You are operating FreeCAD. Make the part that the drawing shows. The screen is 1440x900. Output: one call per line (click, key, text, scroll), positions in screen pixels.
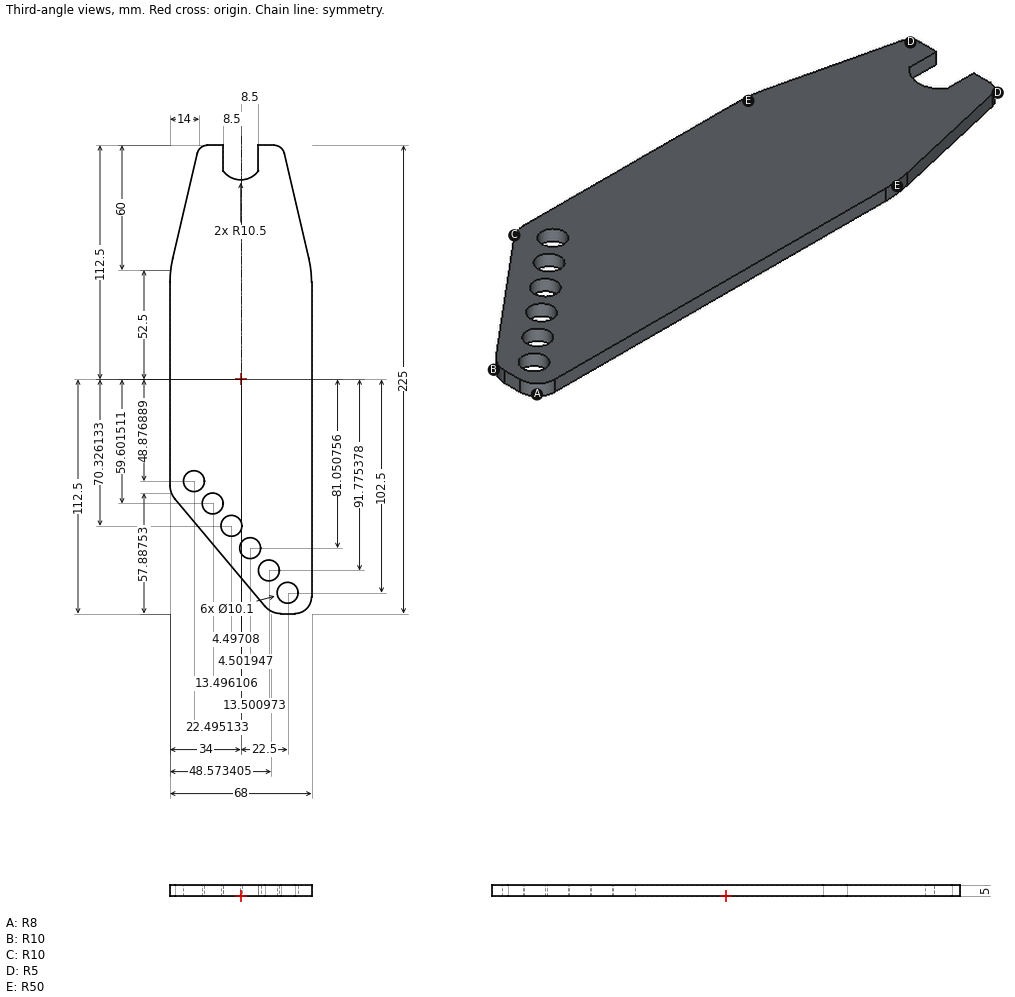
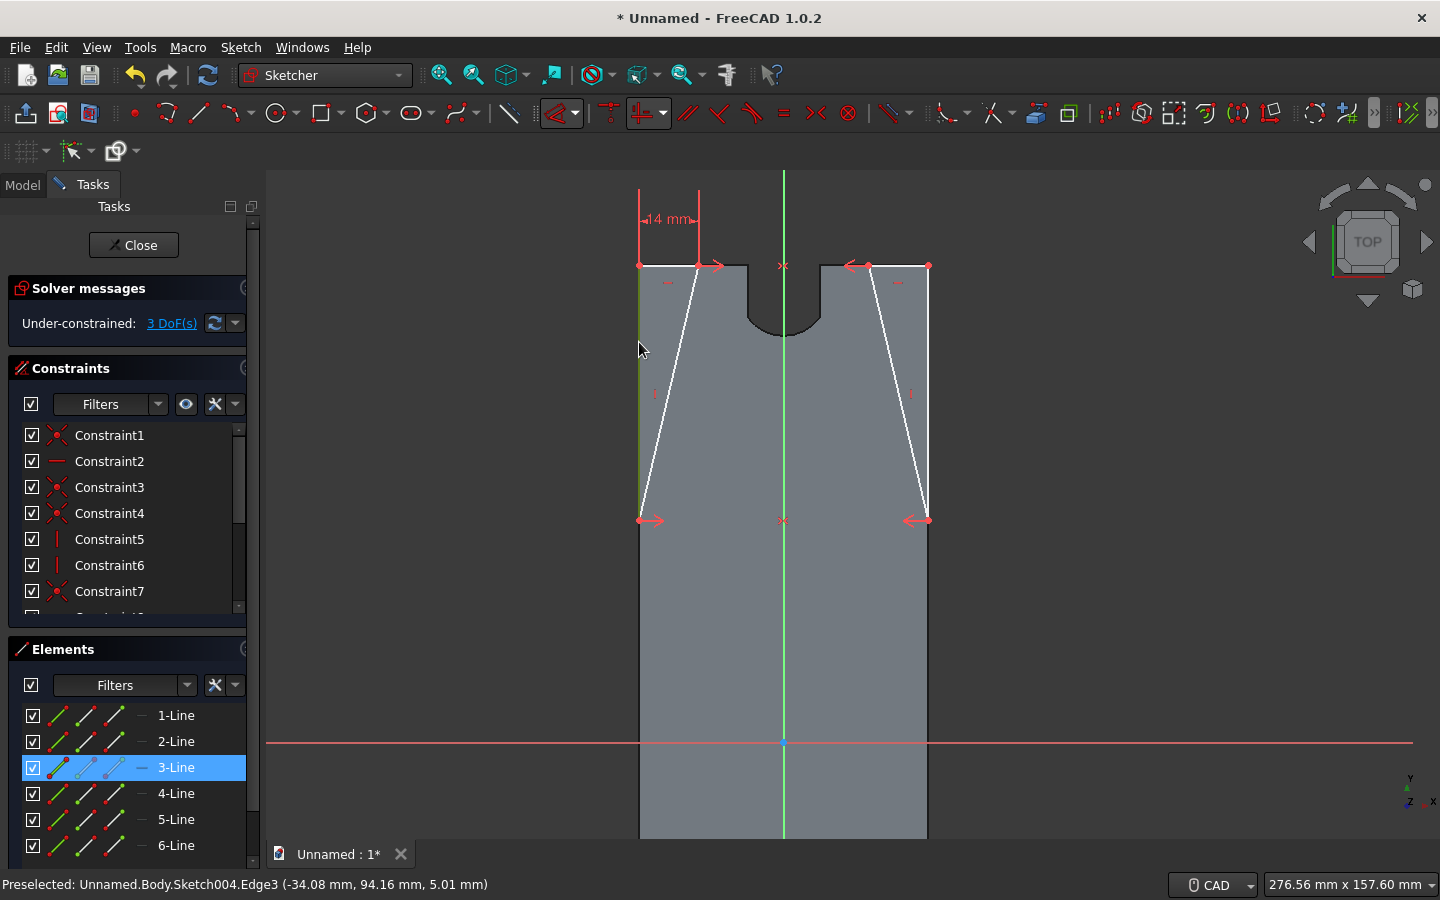
key(i)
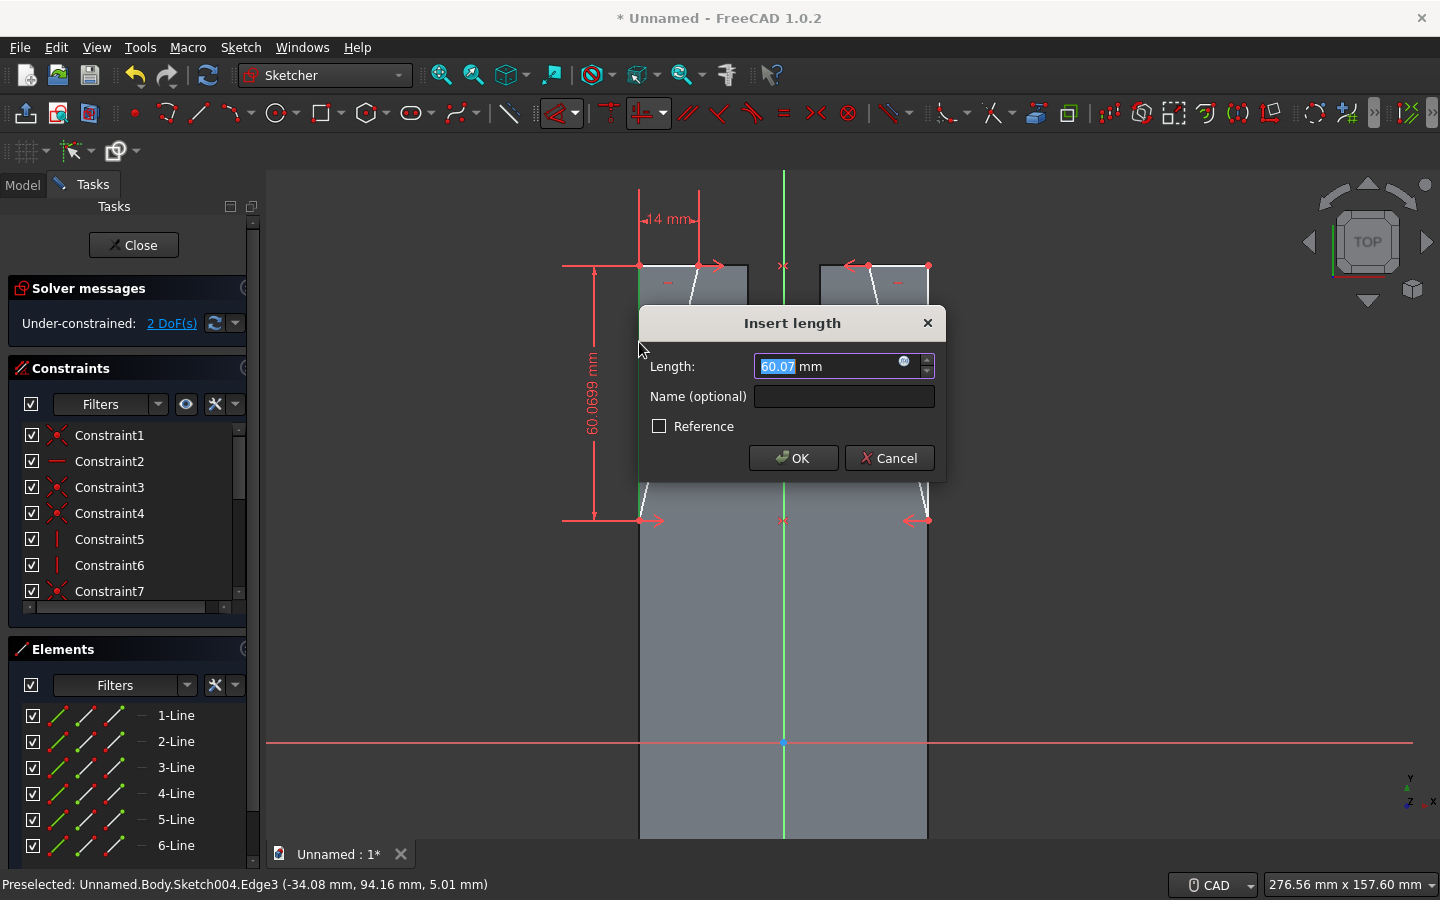
text(60)
key(Return)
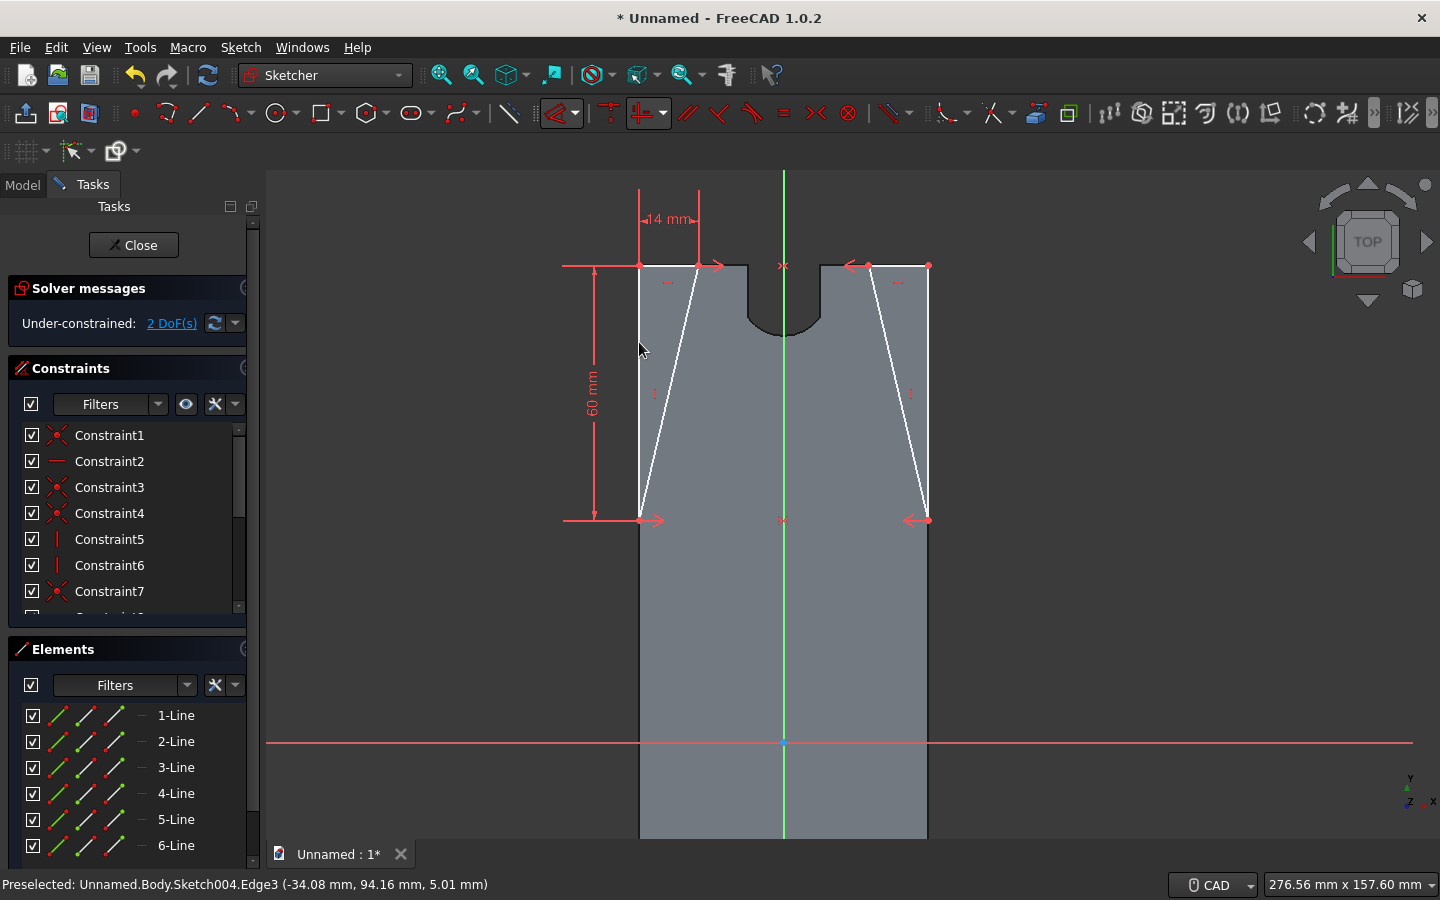
click(639, 521)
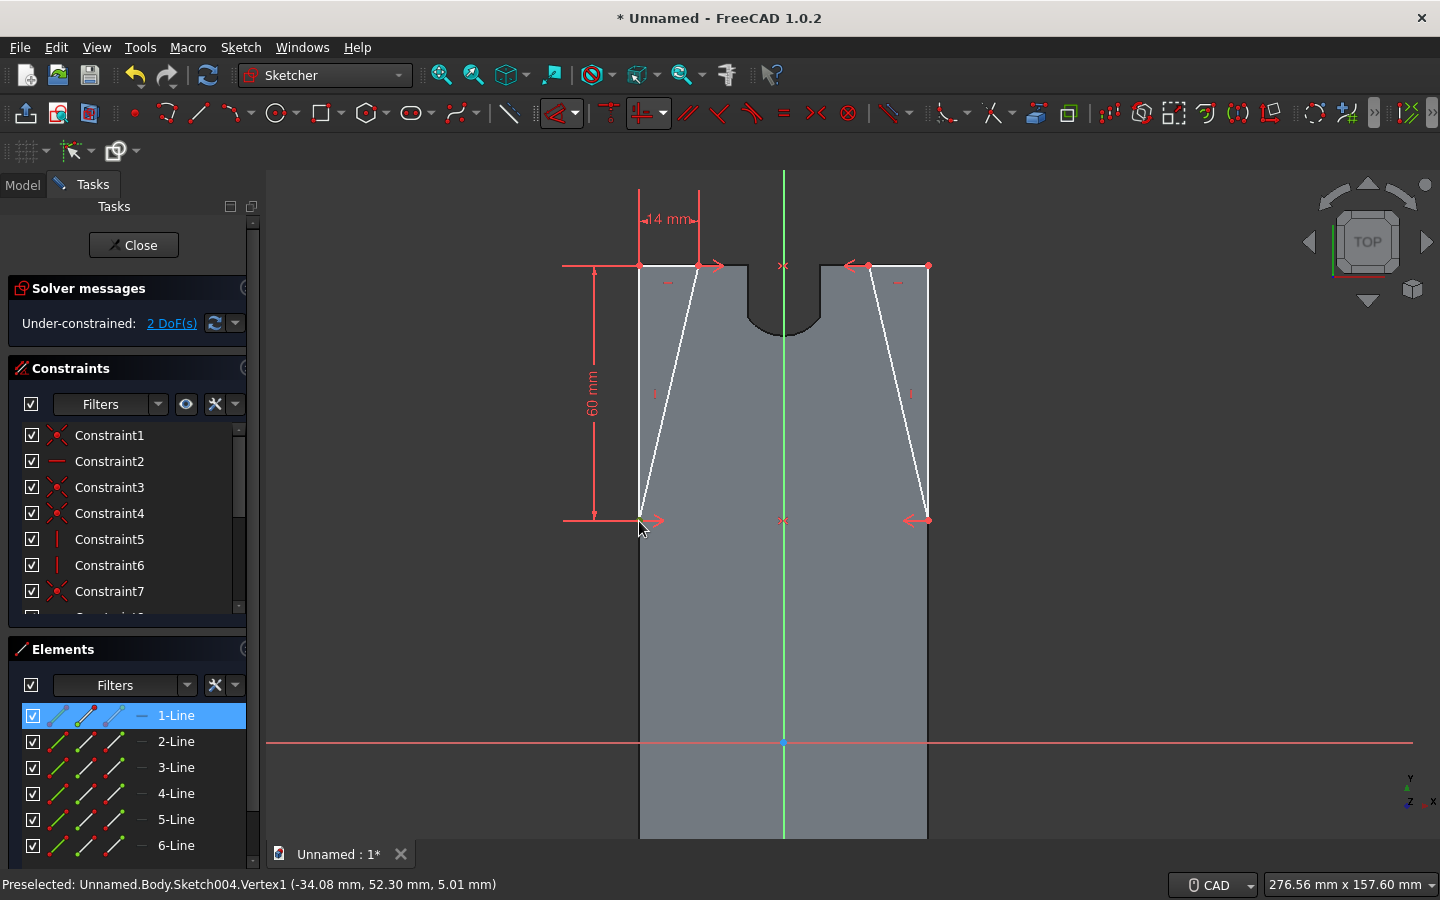
key(l)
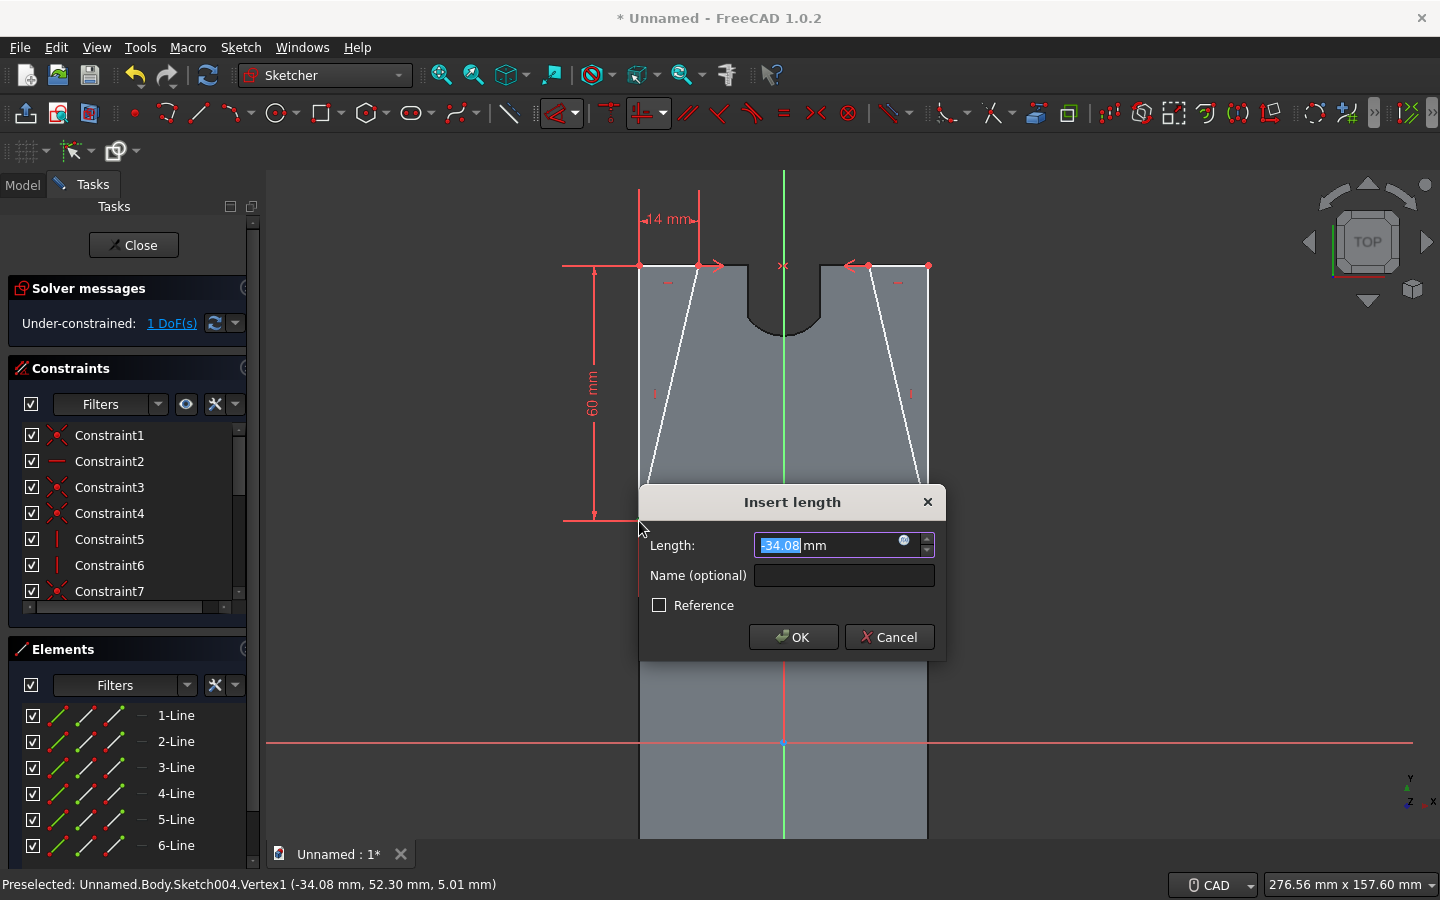
text(-34)
key(Return)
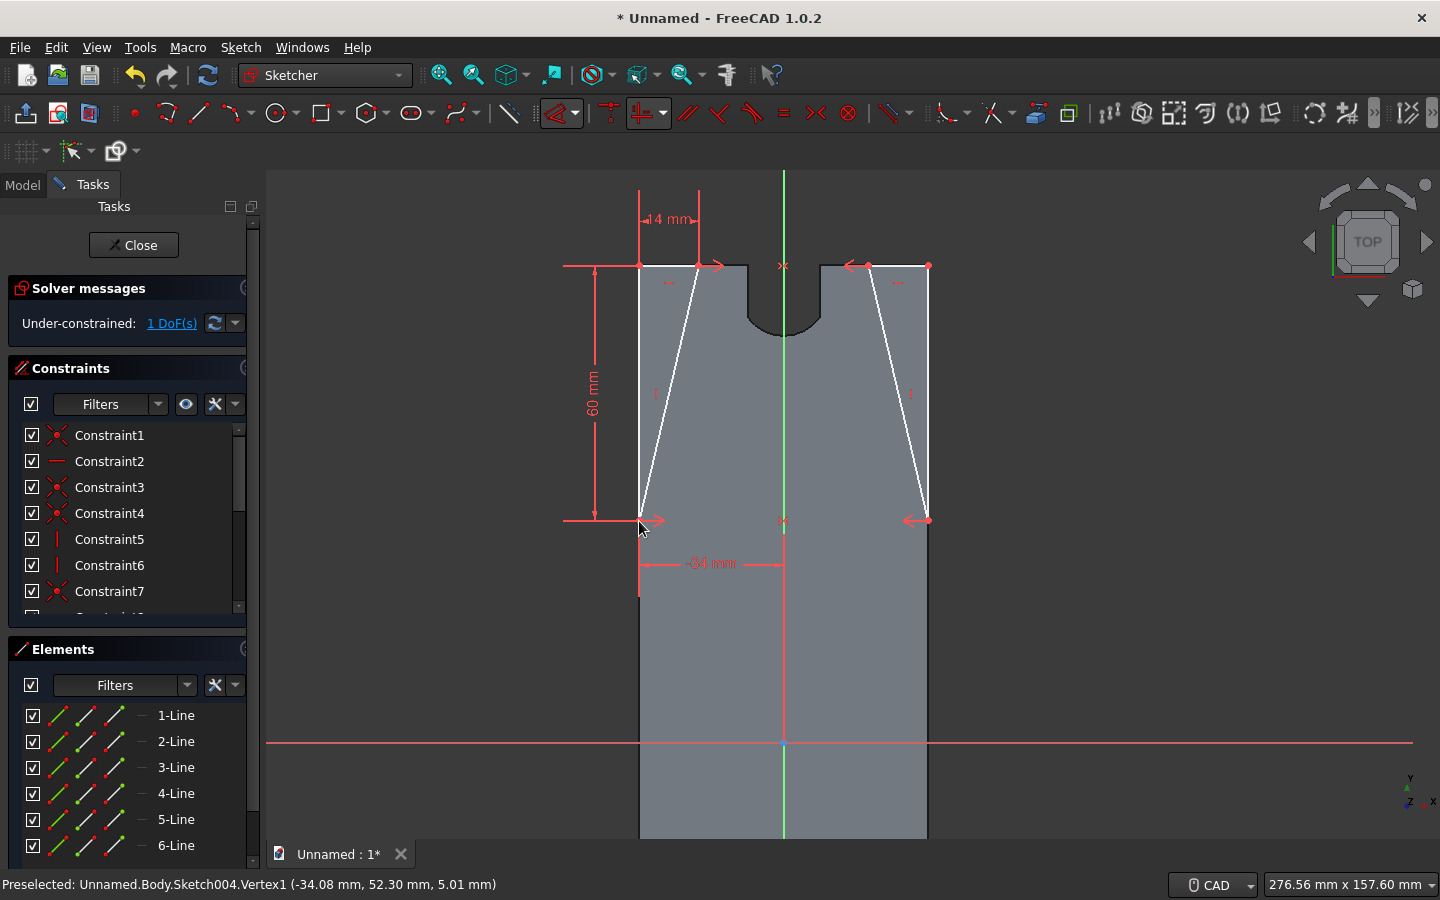
click(639, 521)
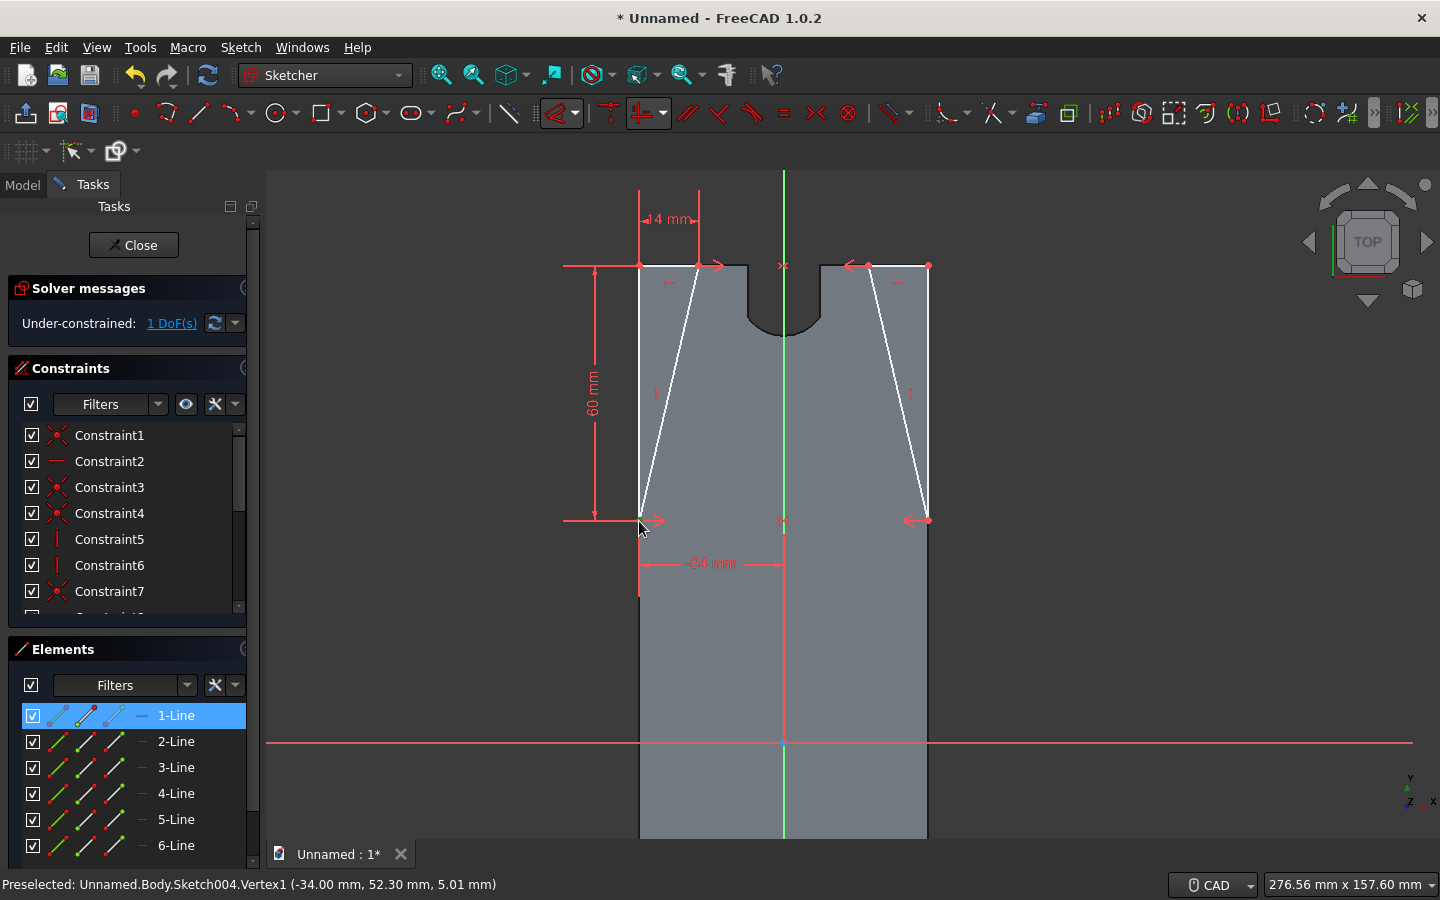
click(578, 114)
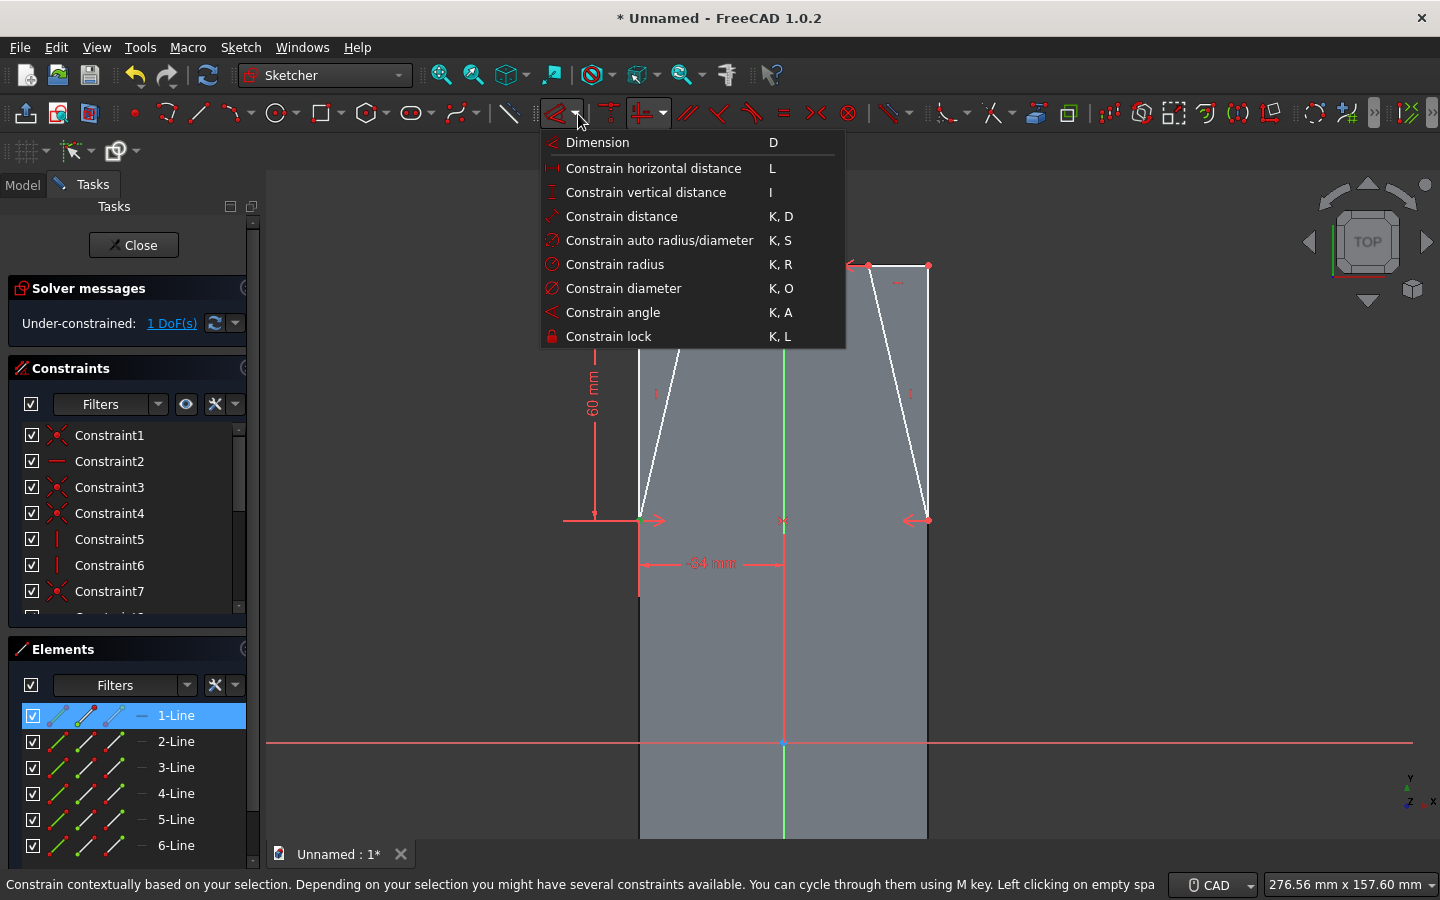
click(693, 192)